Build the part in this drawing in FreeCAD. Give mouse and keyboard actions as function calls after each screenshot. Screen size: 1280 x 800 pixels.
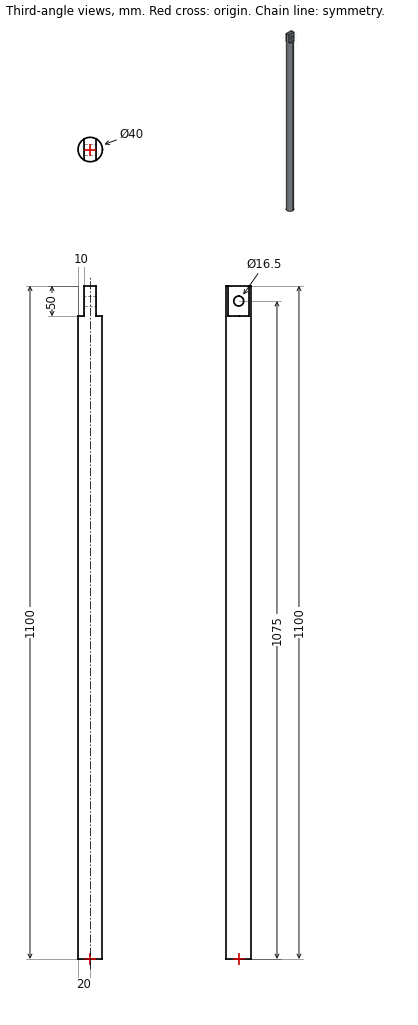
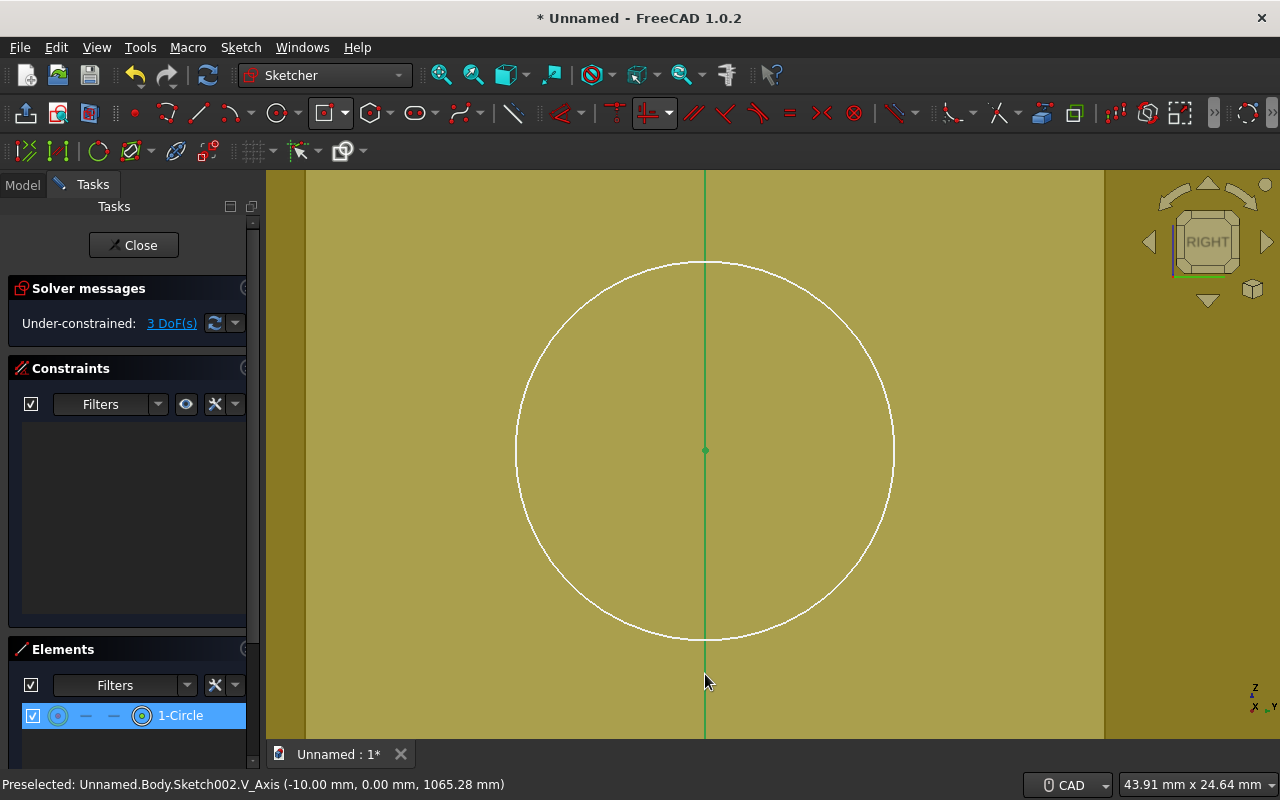
click(616, 114)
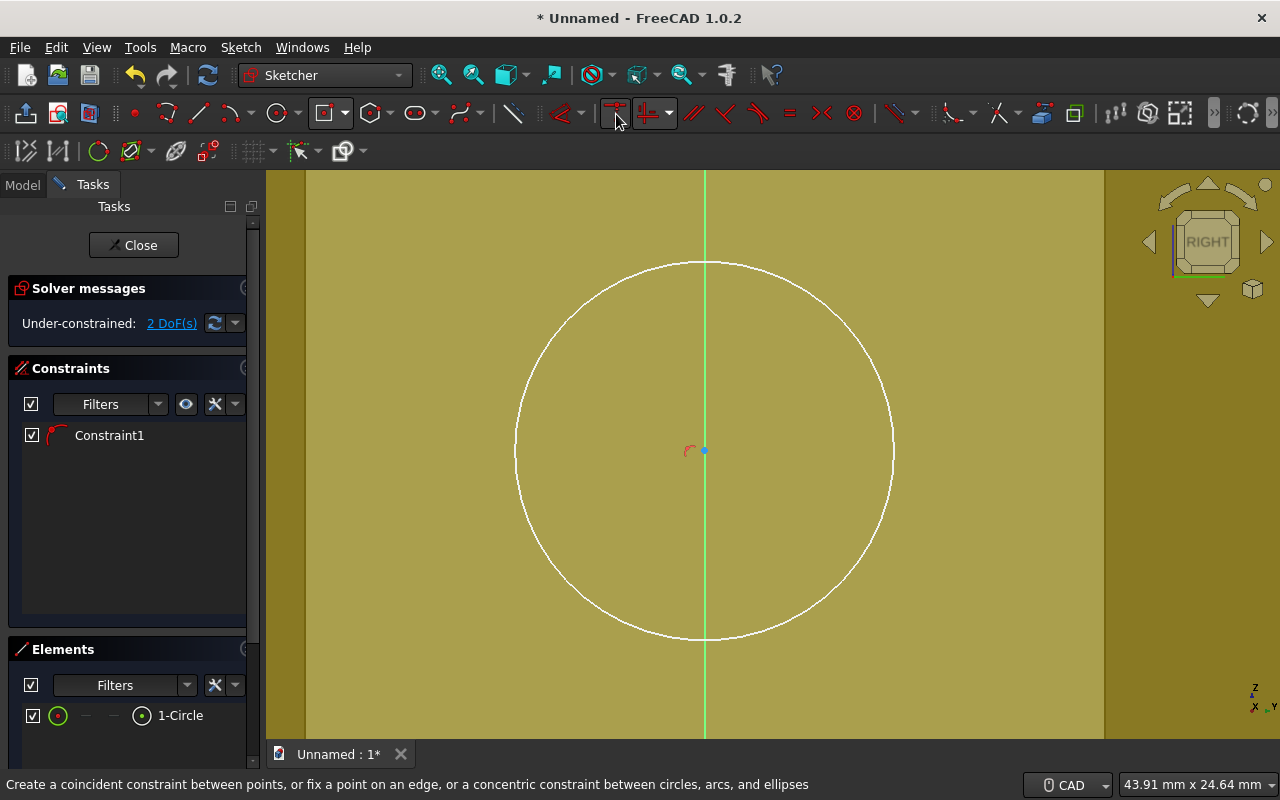
click(560, 114)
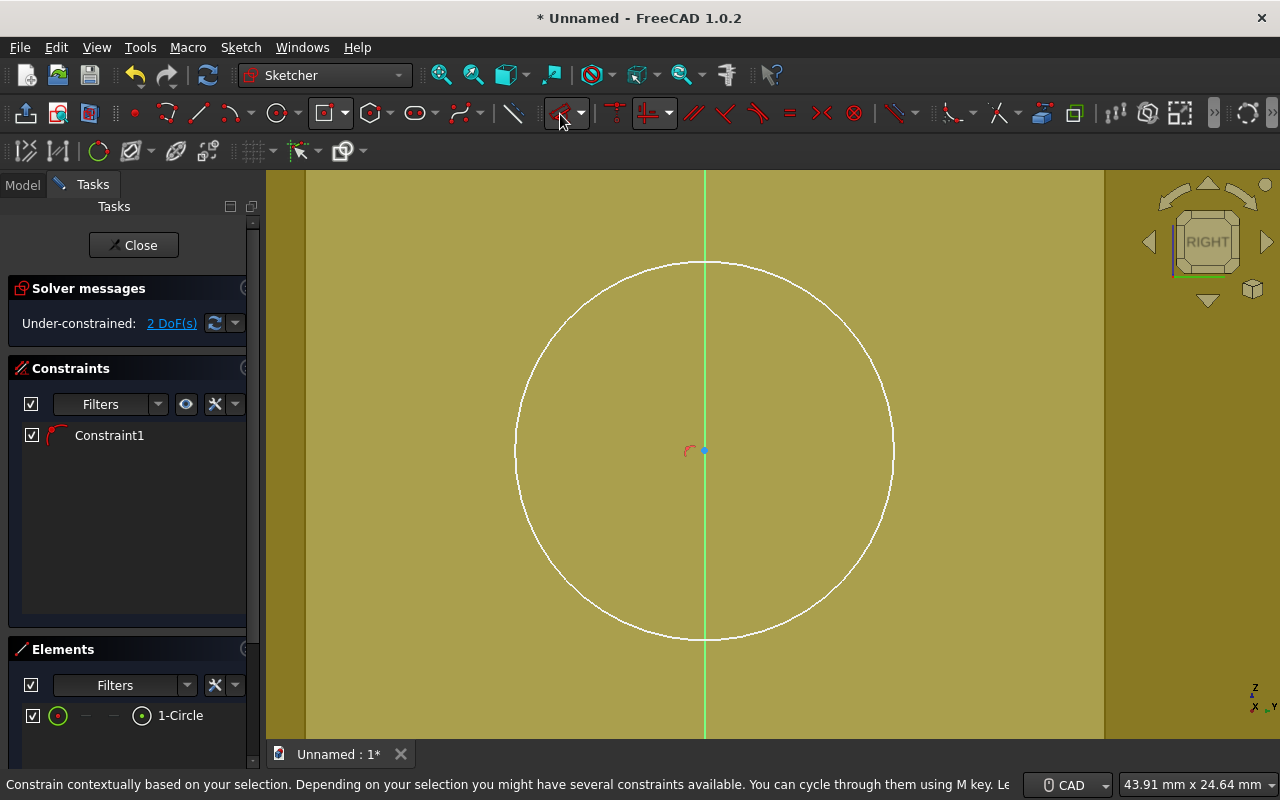
click(838, 317)
click(861, 294)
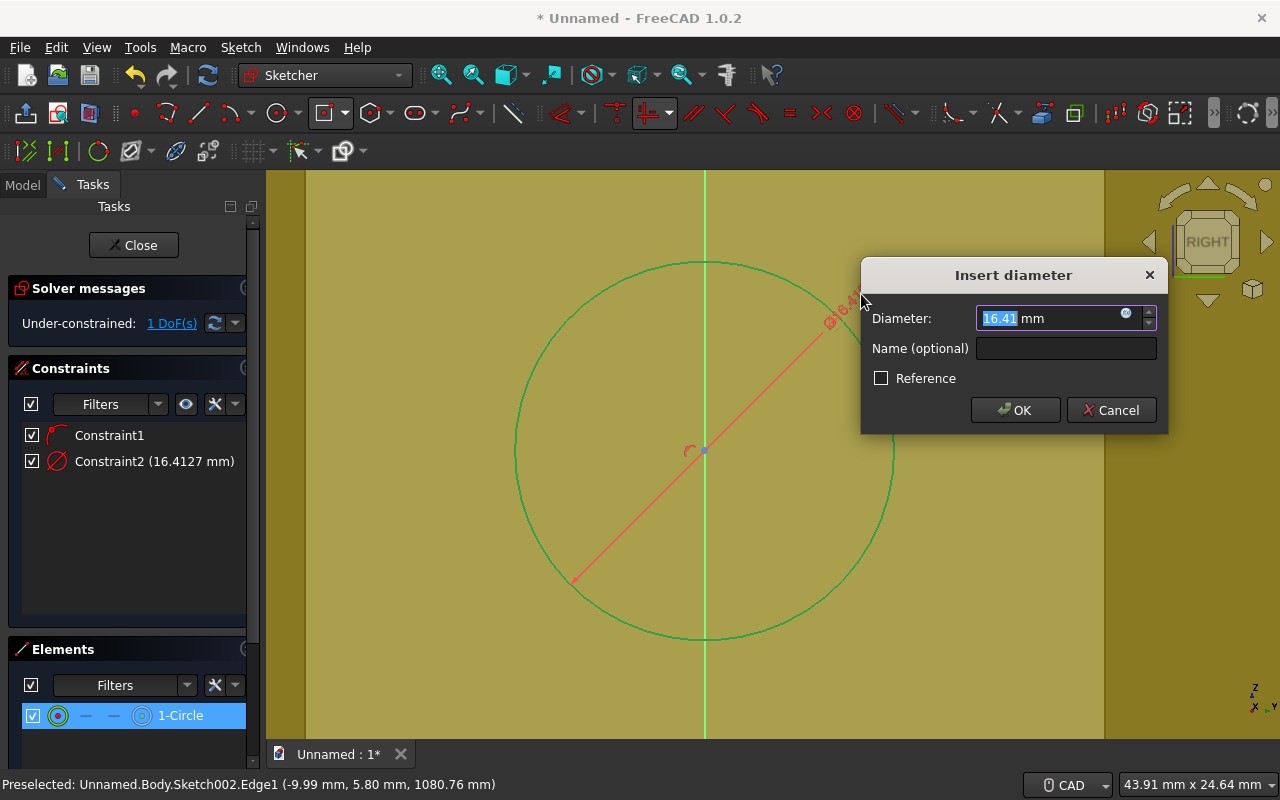
text(16.5)
key(Return)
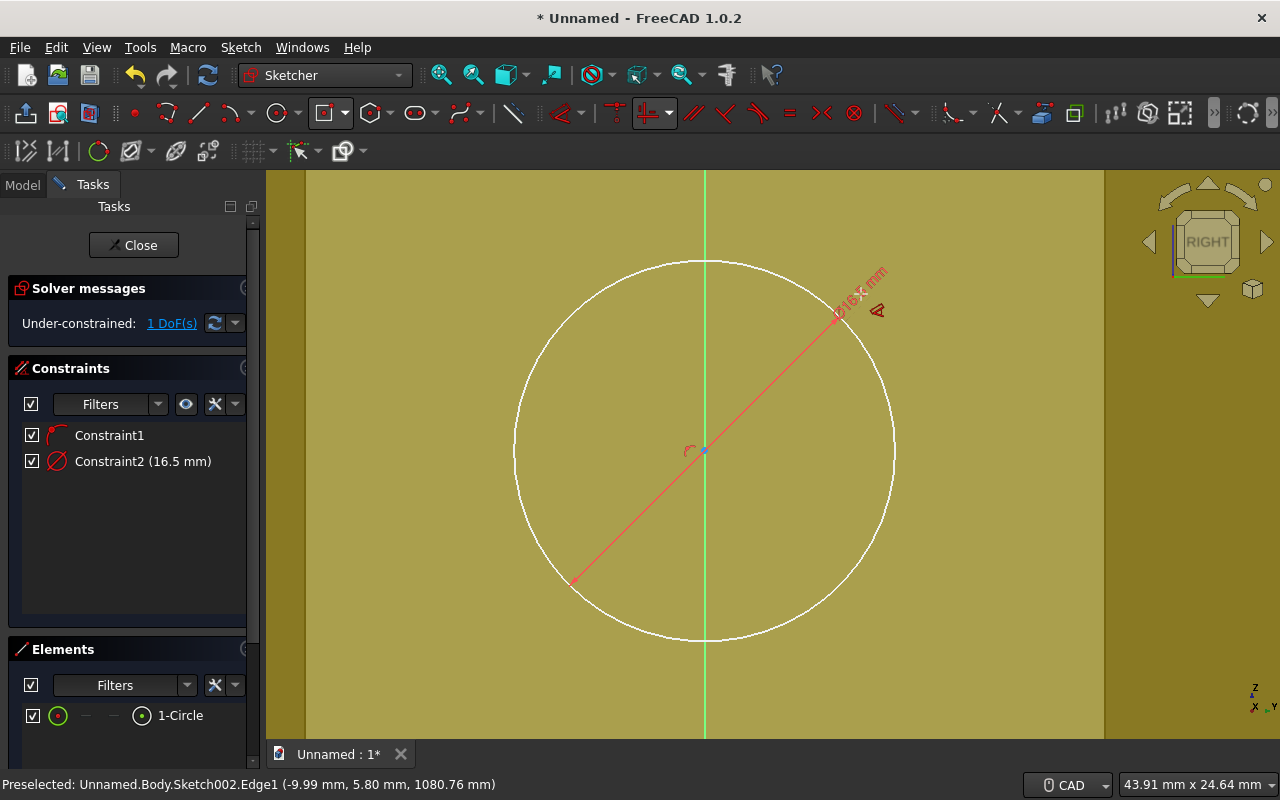
click(705, 451)
click(739, 581)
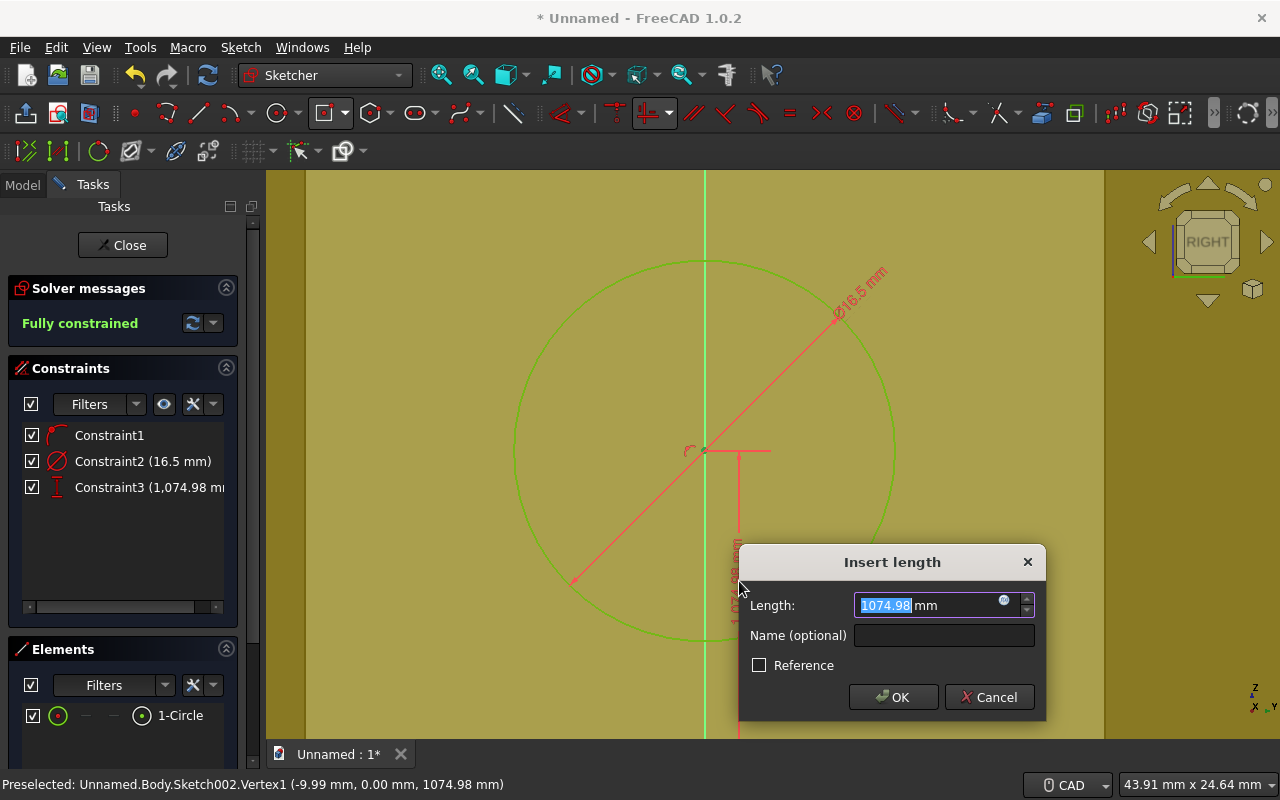
text(1075)
key(Return)
key(Escape)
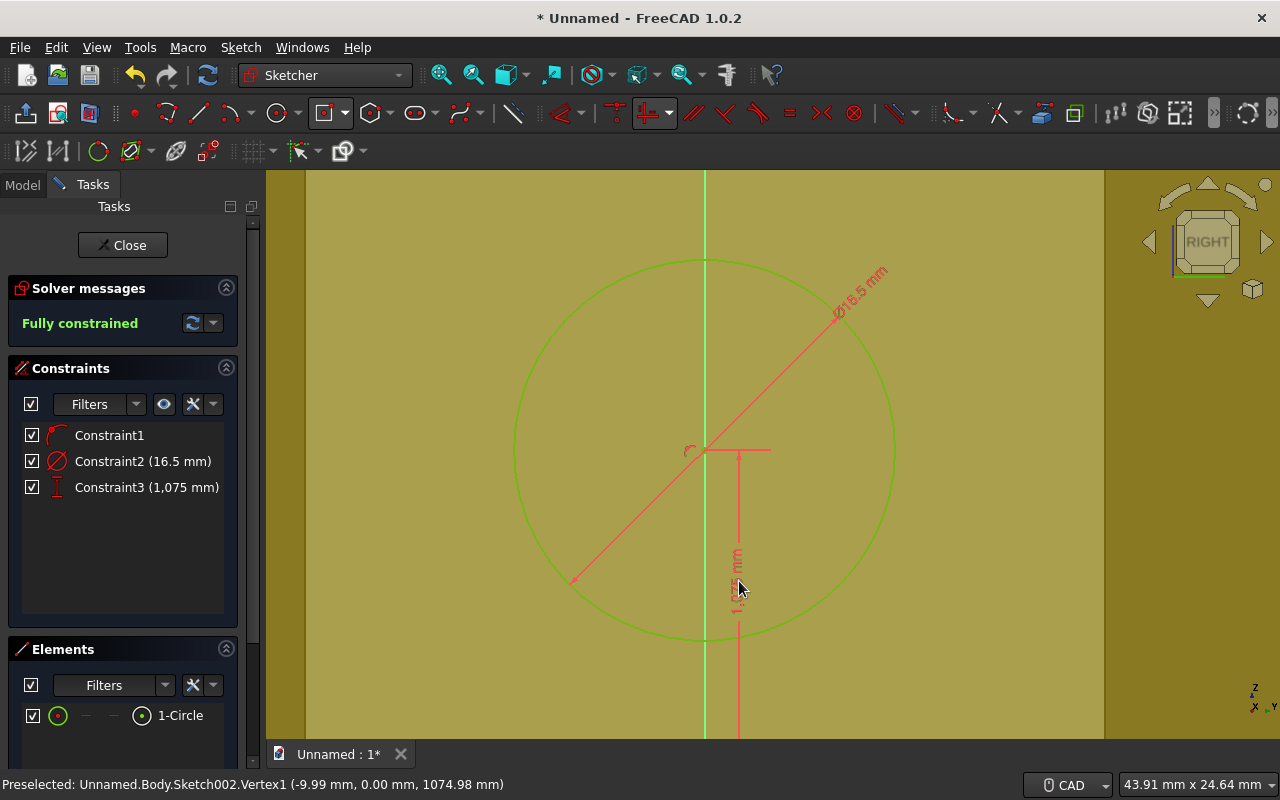
click(123, 245)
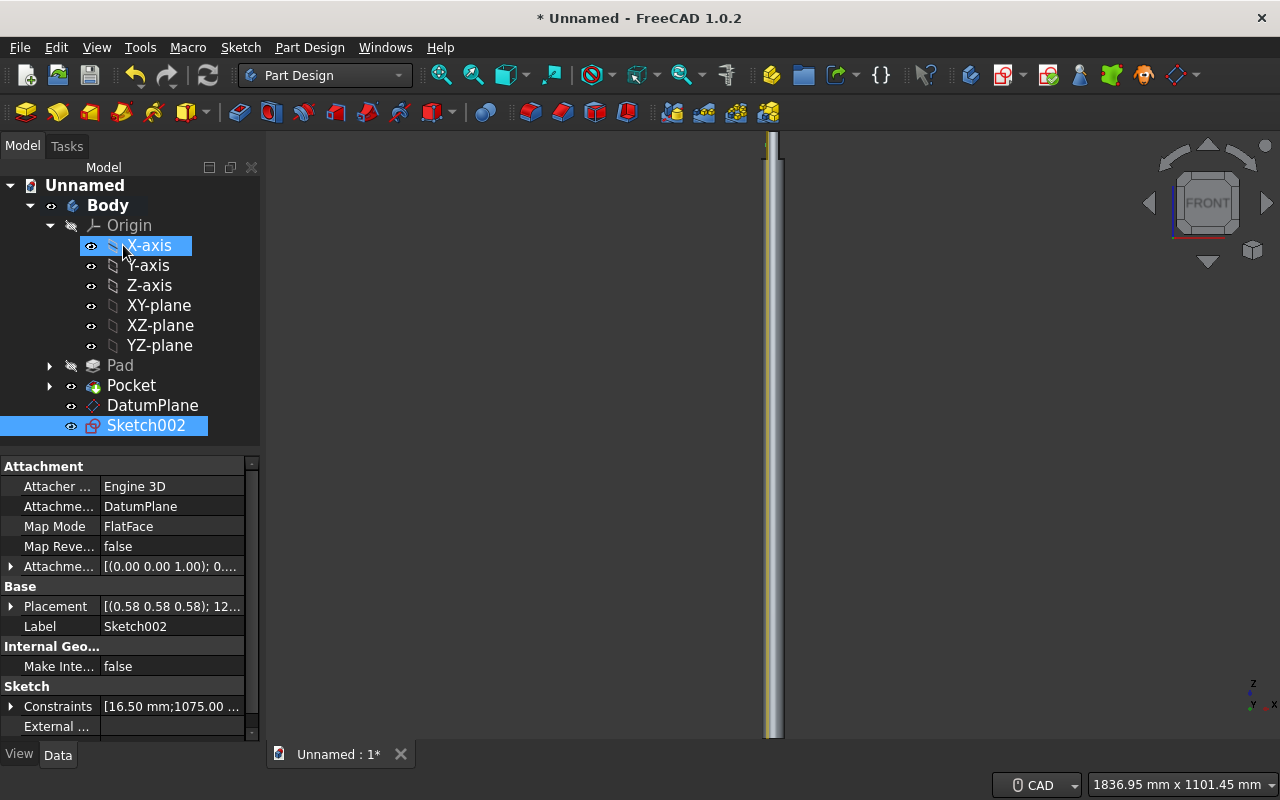
click(240, 112)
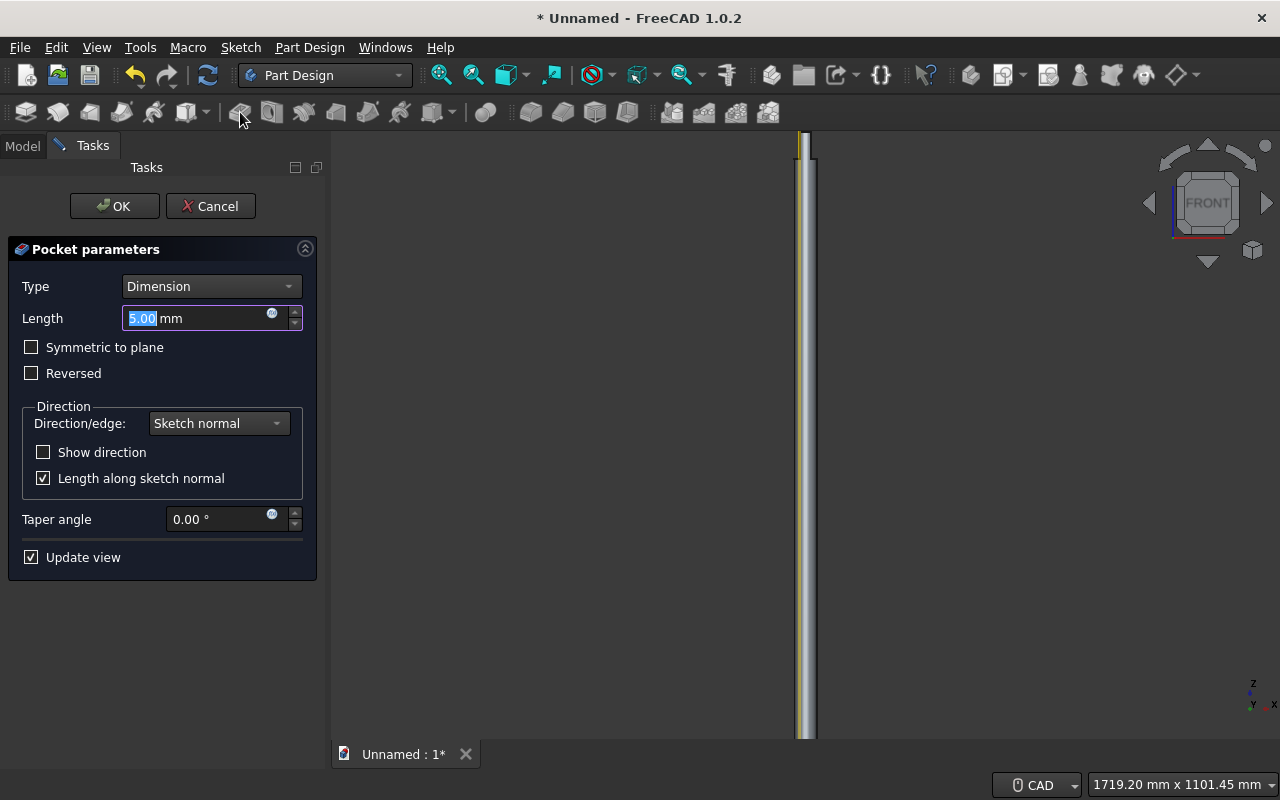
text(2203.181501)
key(Tab)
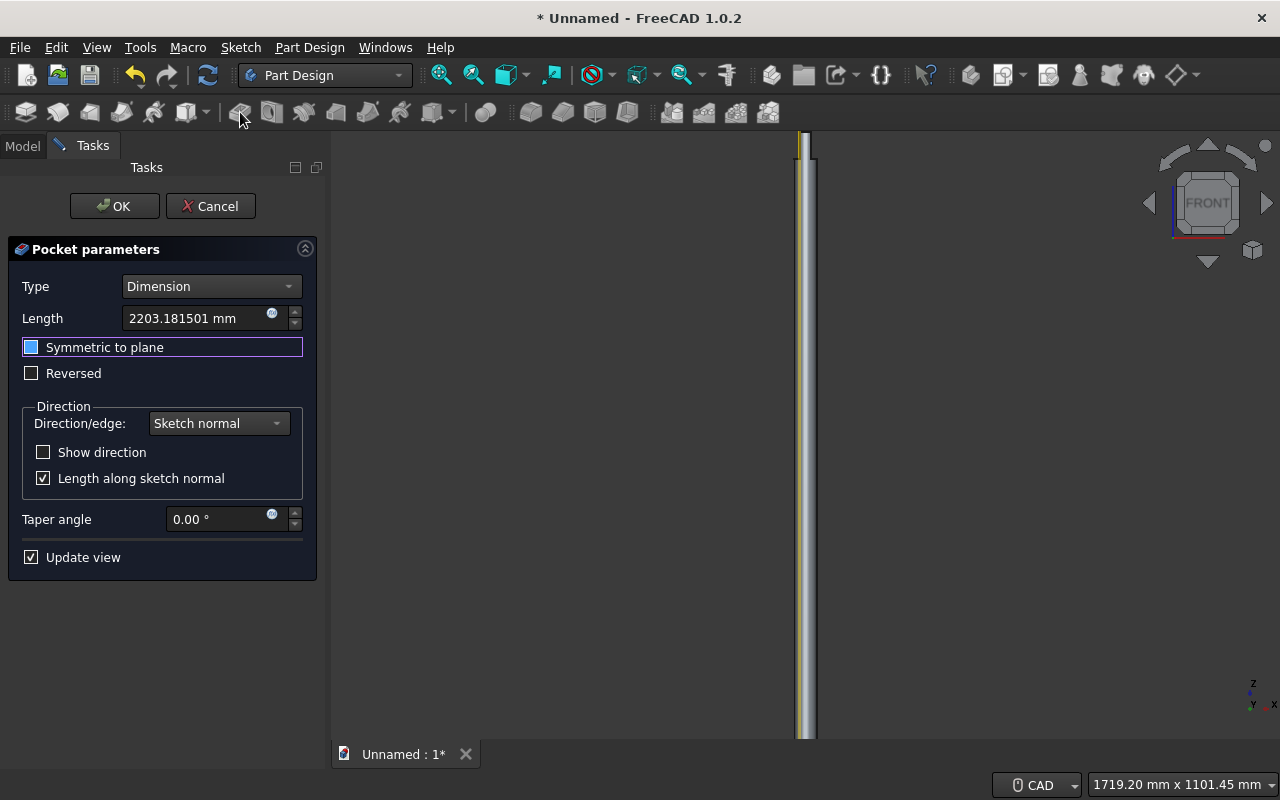
click(30, 347)